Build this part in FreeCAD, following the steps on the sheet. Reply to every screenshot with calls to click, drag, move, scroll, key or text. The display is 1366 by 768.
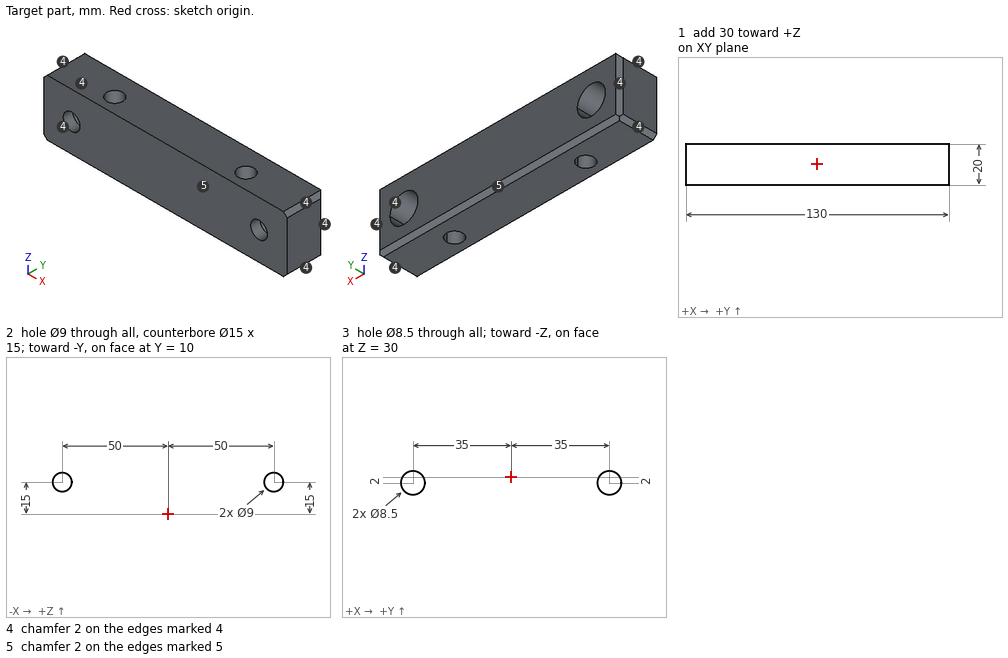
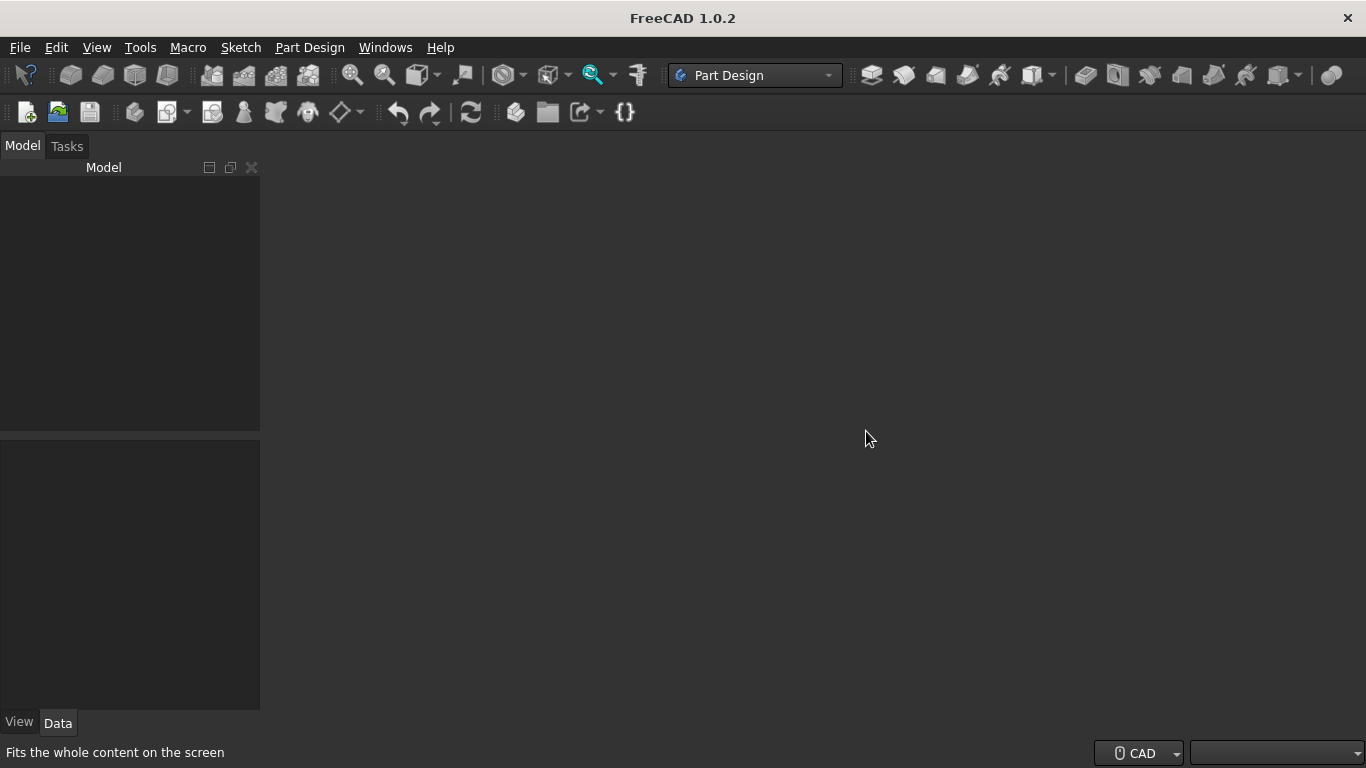
click(26, 112)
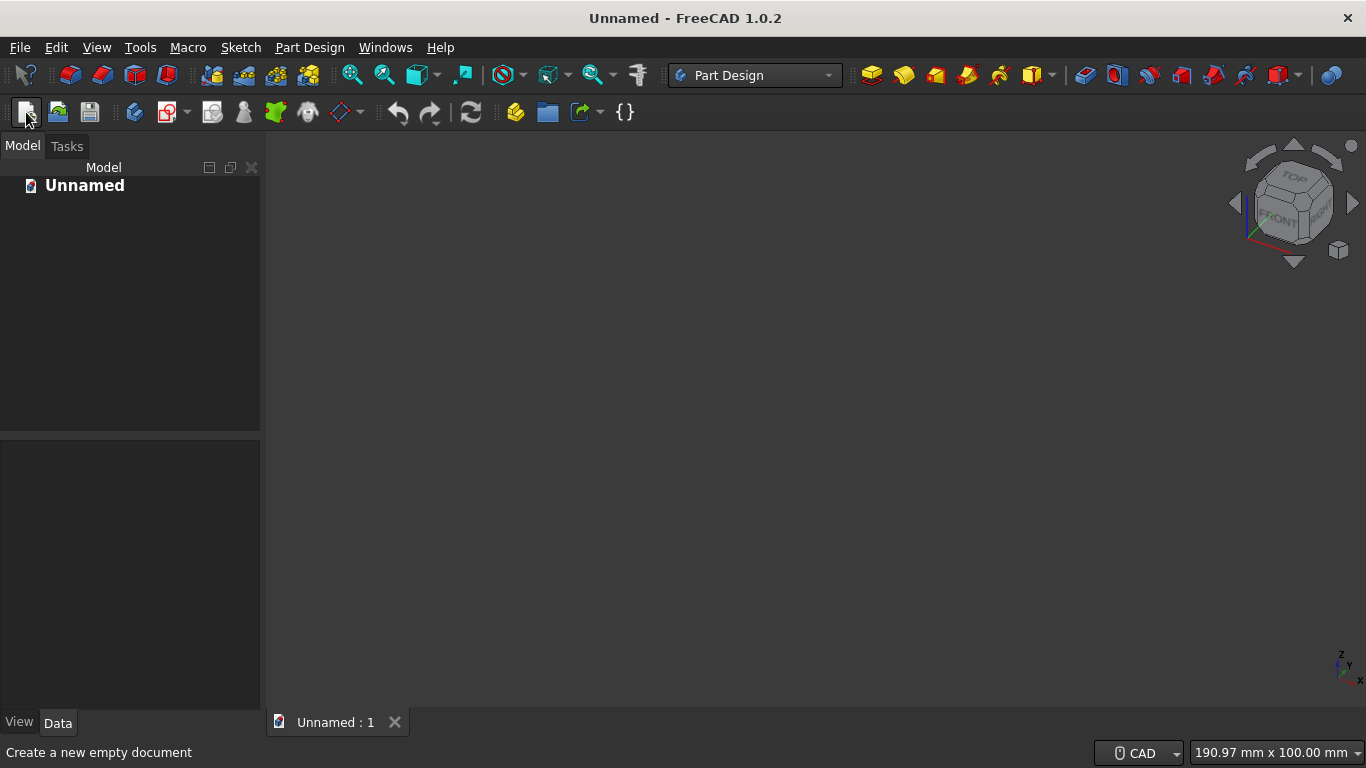
click(168, 112)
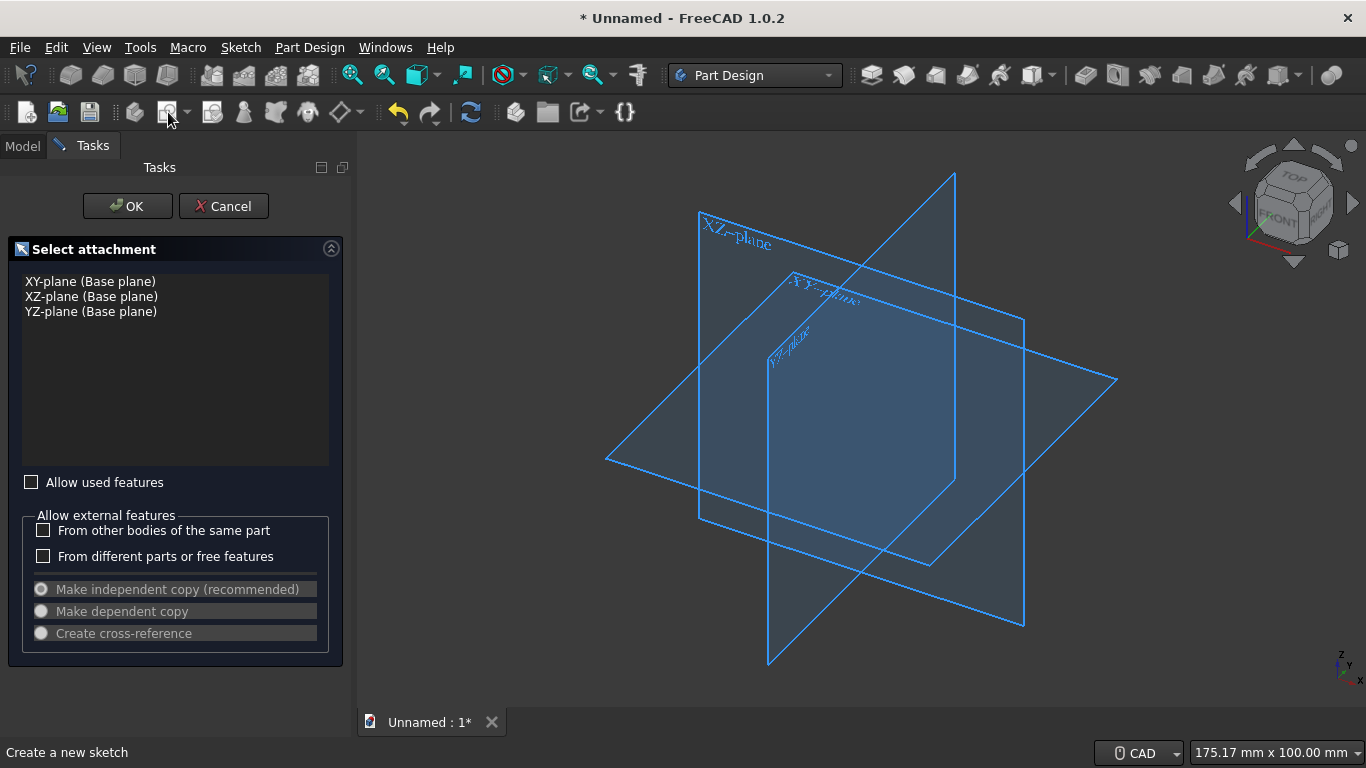
click(82, 282)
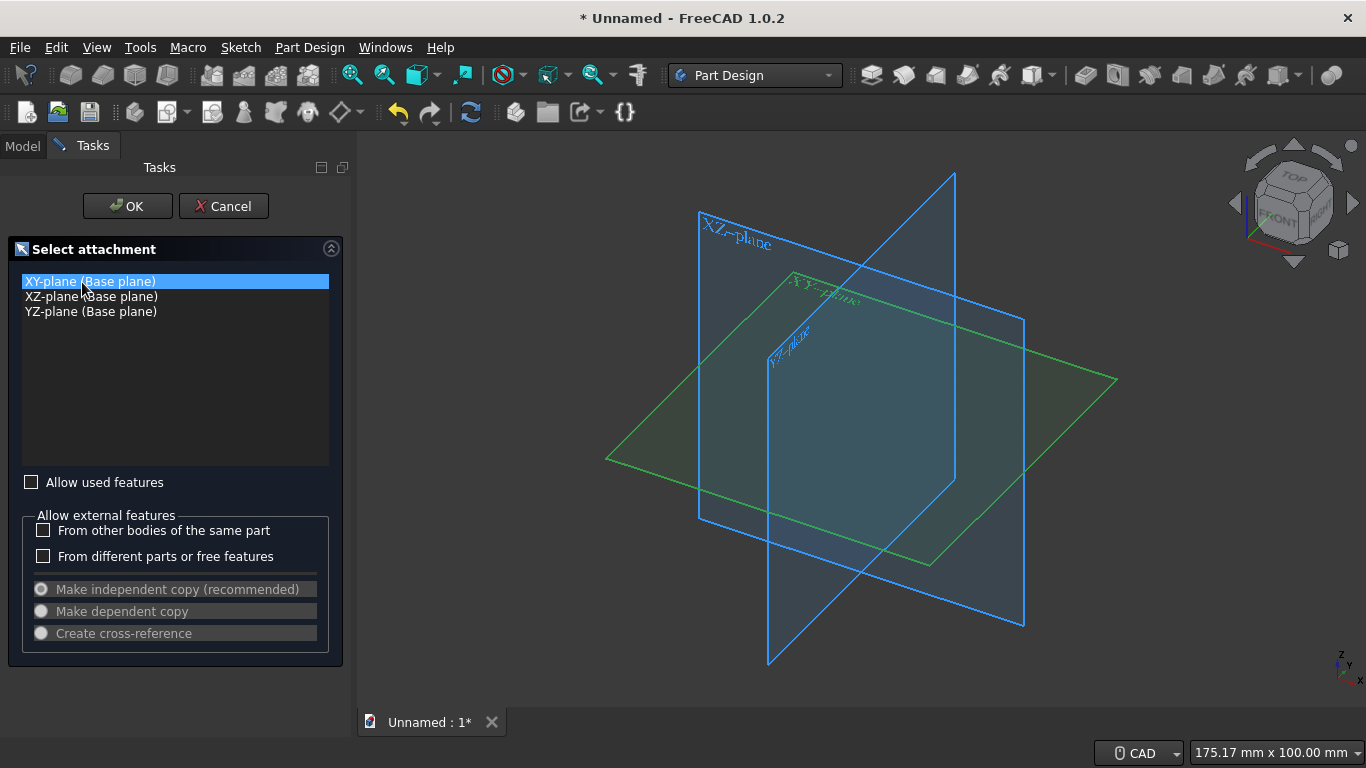
click(128, 206)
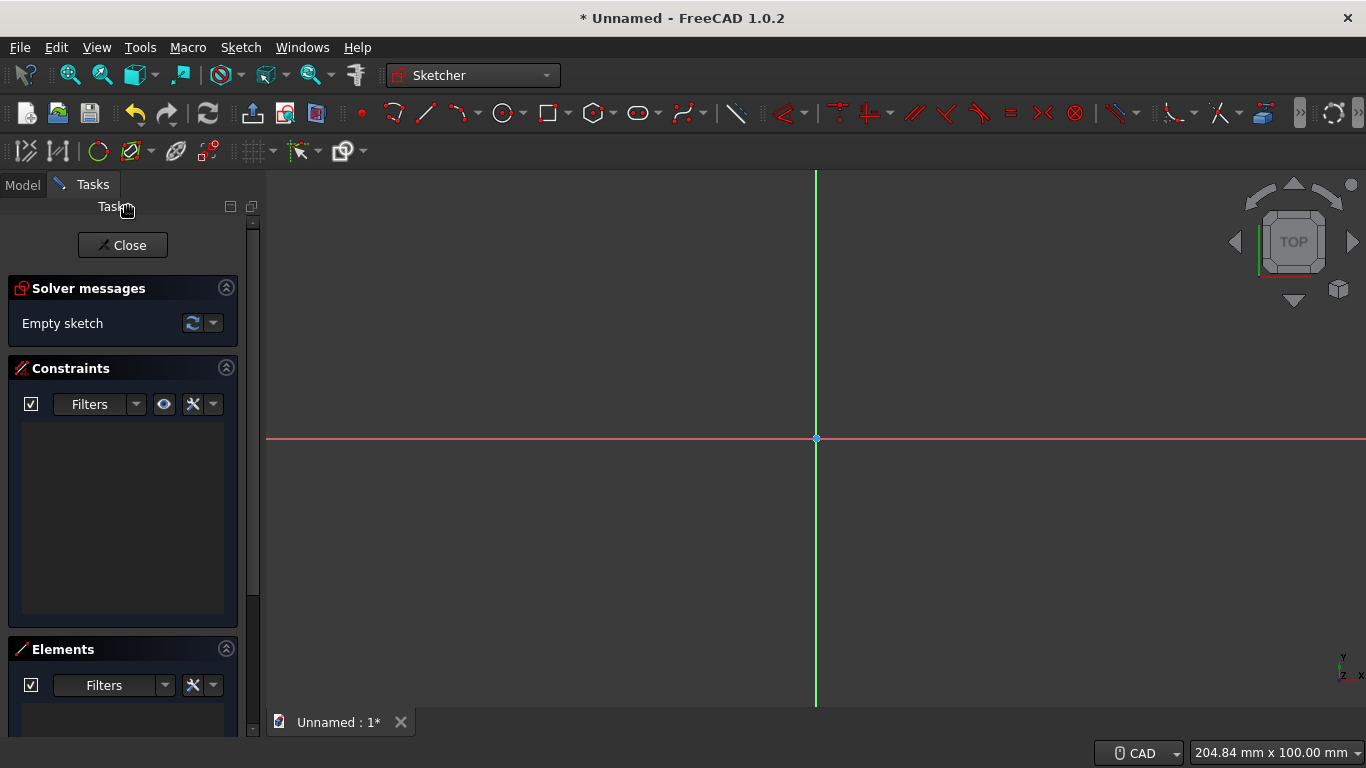
key(g)
key(v)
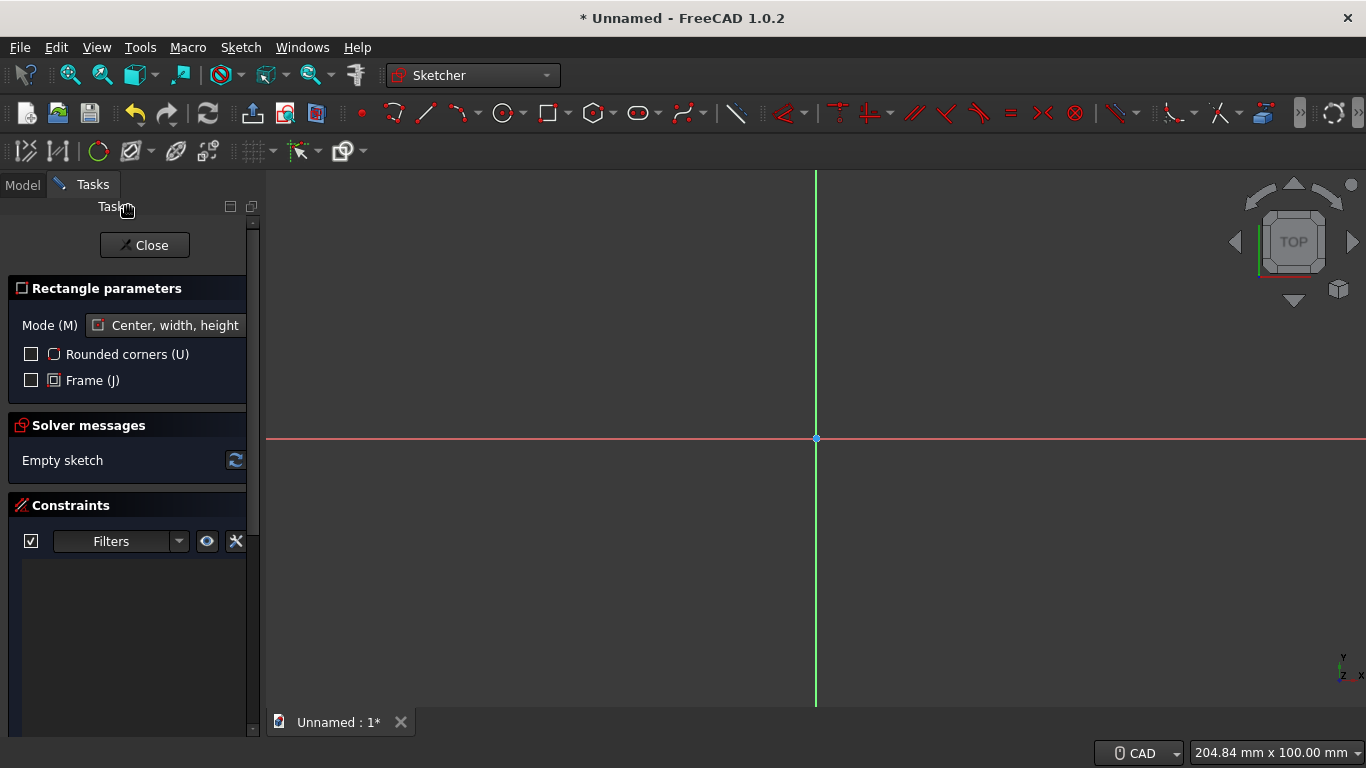
click(816, 438)
move(1165, 385)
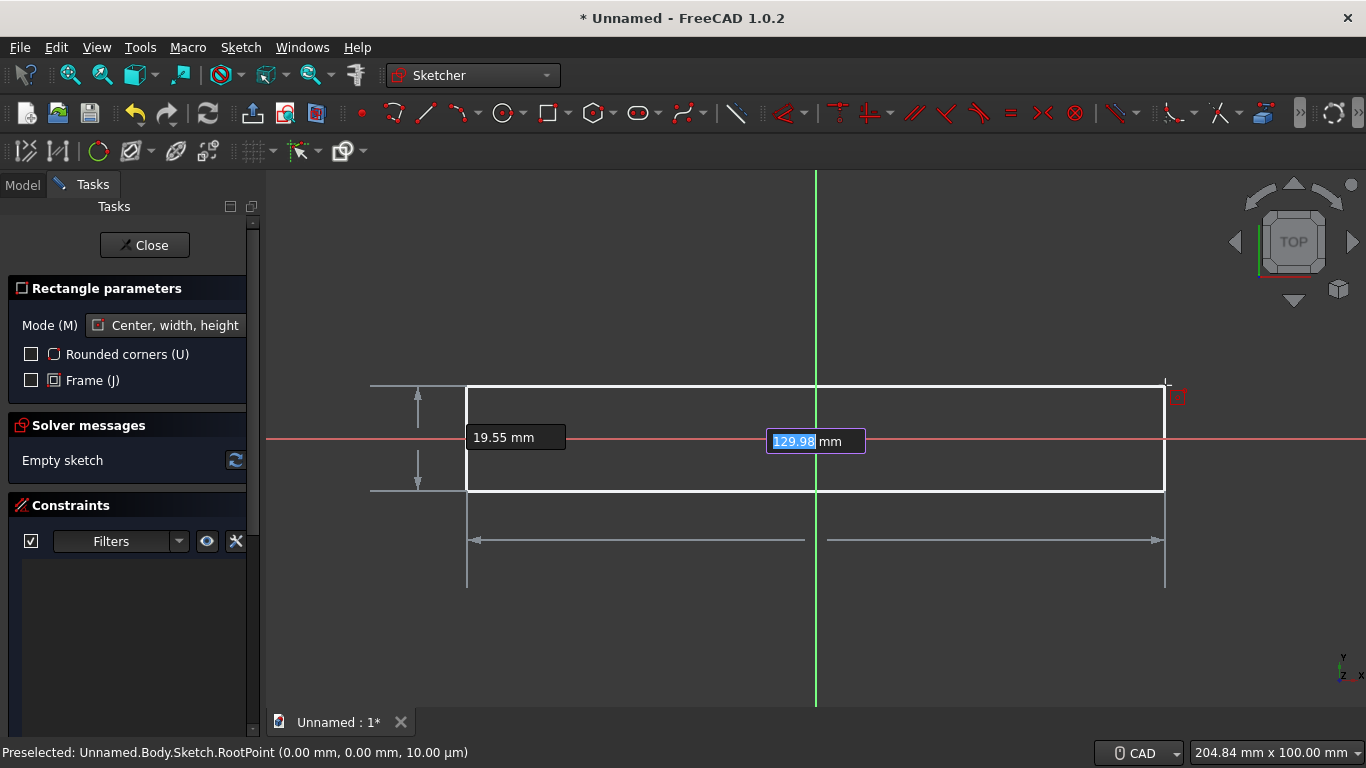
text(130)
key(Tab)
text(20)
key(Return)
key(Escape)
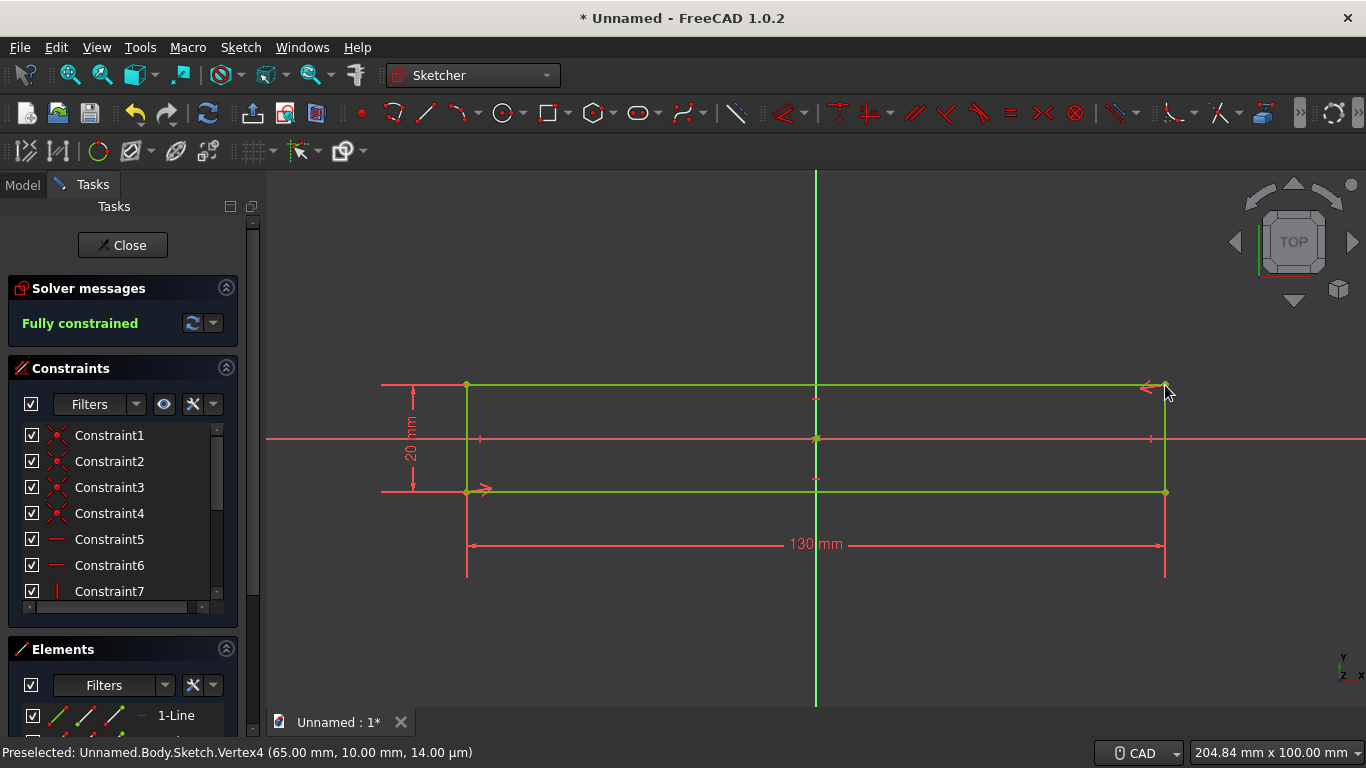
click(123, 245)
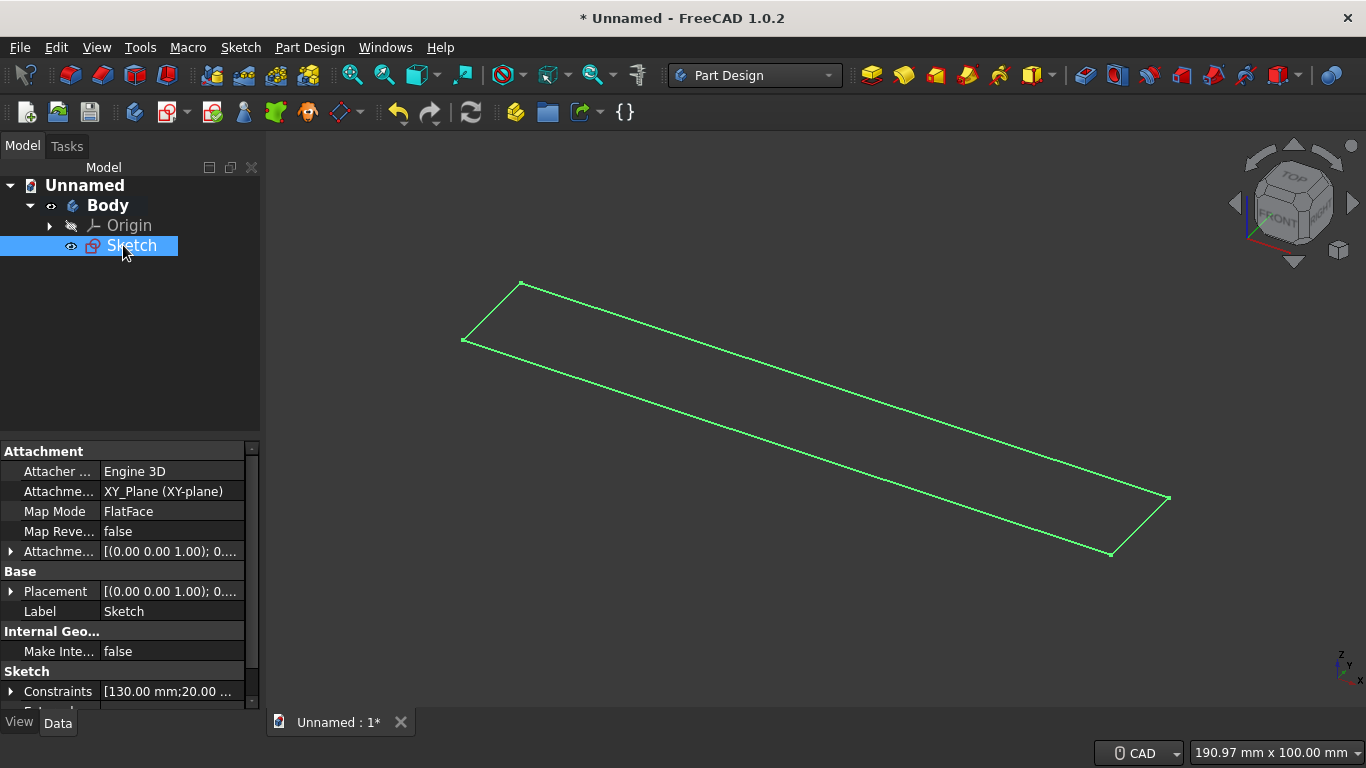
click(872, 76)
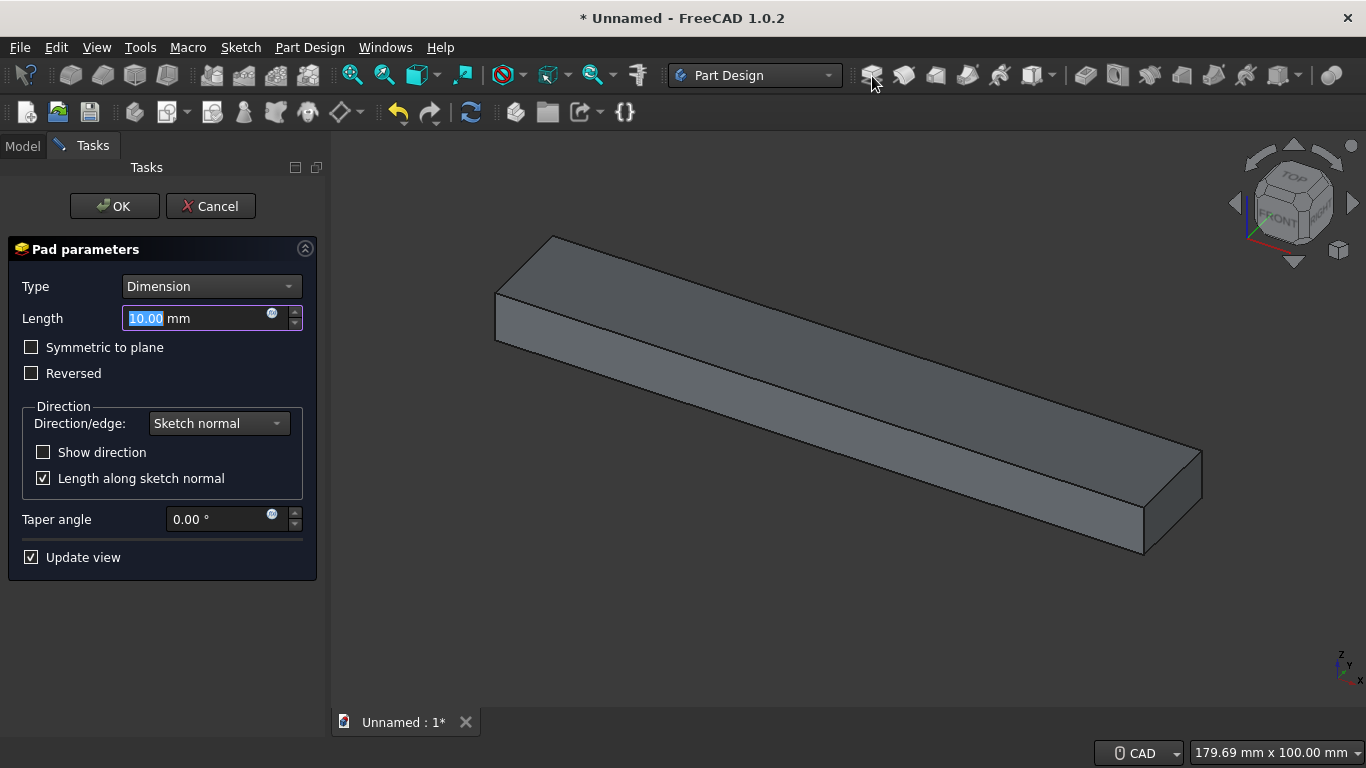
text(30)
key(Tab)